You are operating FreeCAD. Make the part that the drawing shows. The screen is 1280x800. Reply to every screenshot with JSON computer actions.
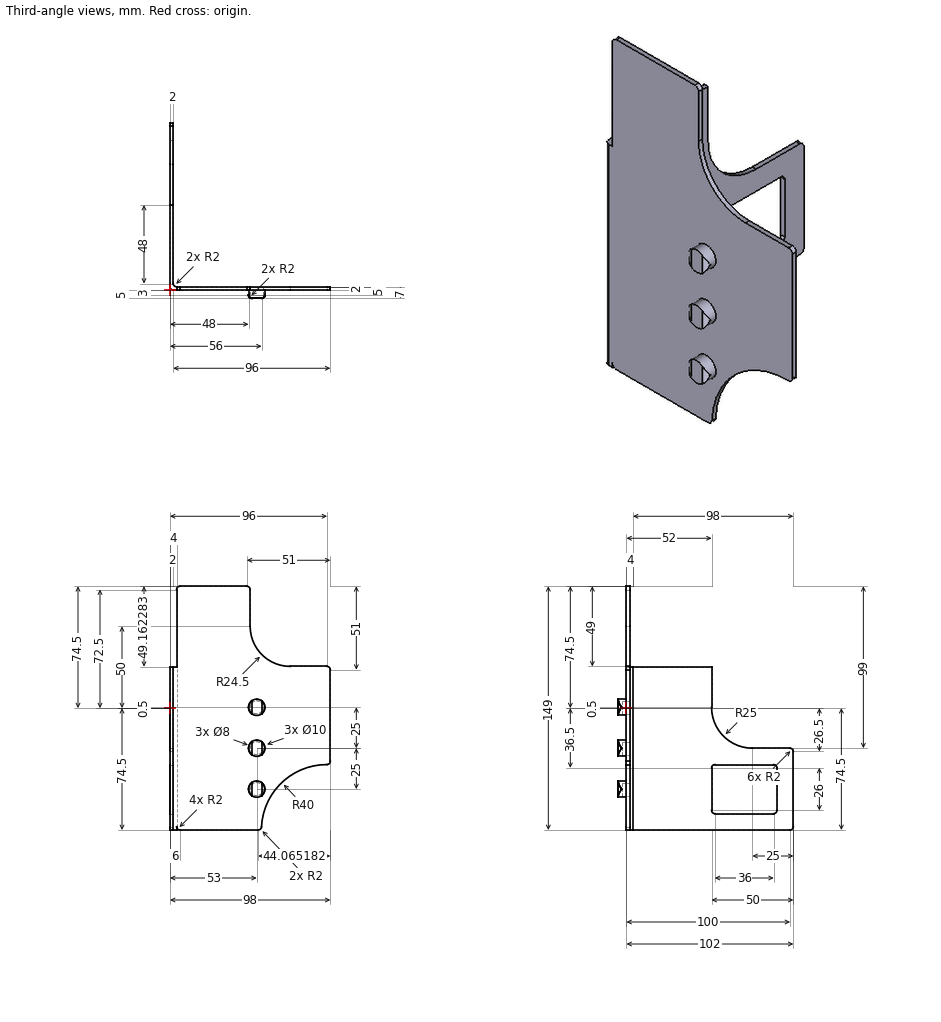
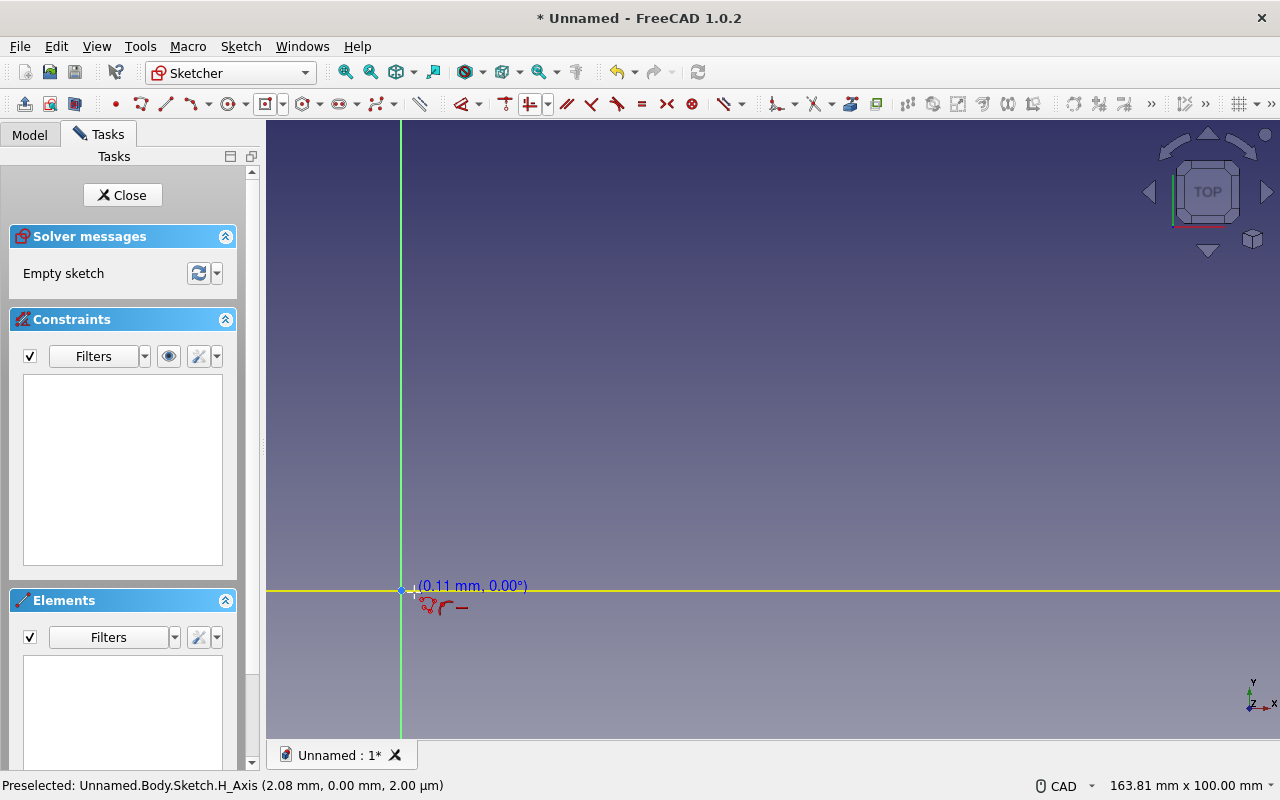
{"action": "left_click", "coordinate": [1008, 582]}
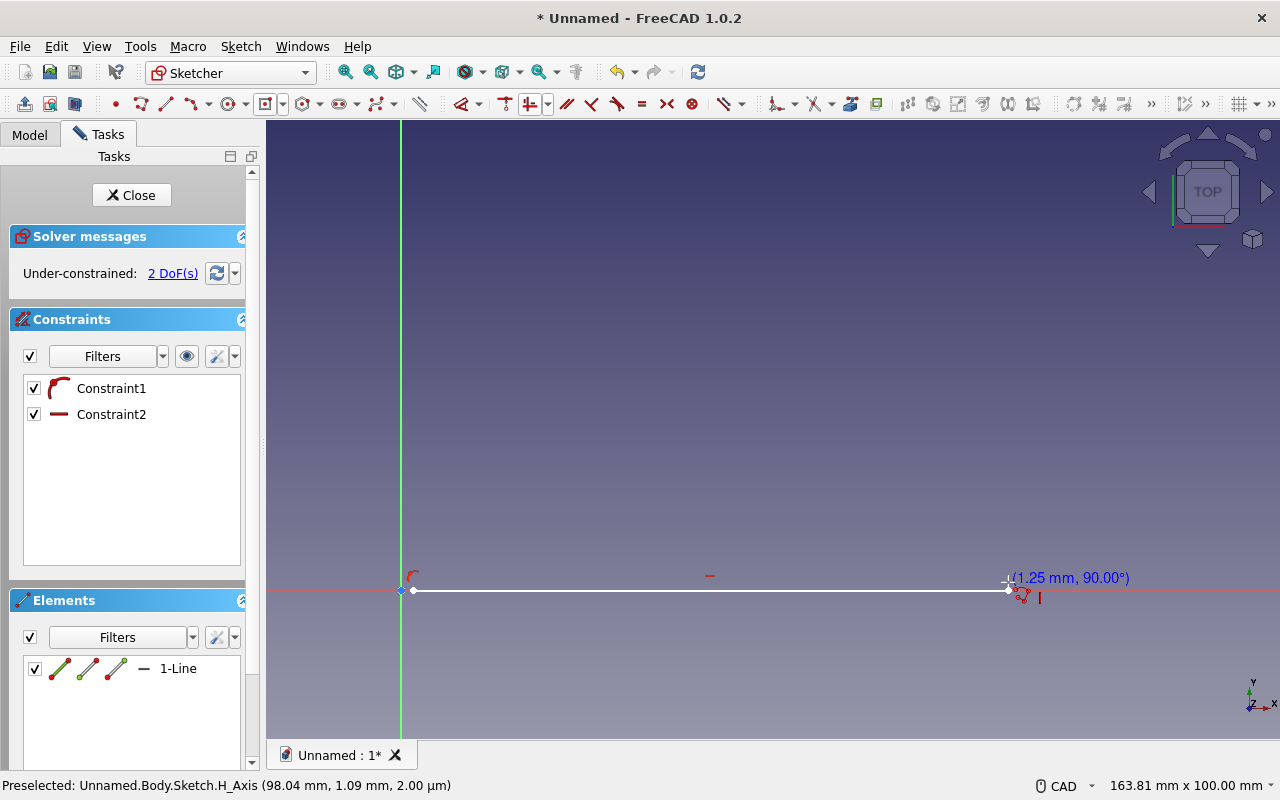
{"action": "scroll", "coordinate": [1008, 578], "scroll_direction": "up", "scroll_amount": 2}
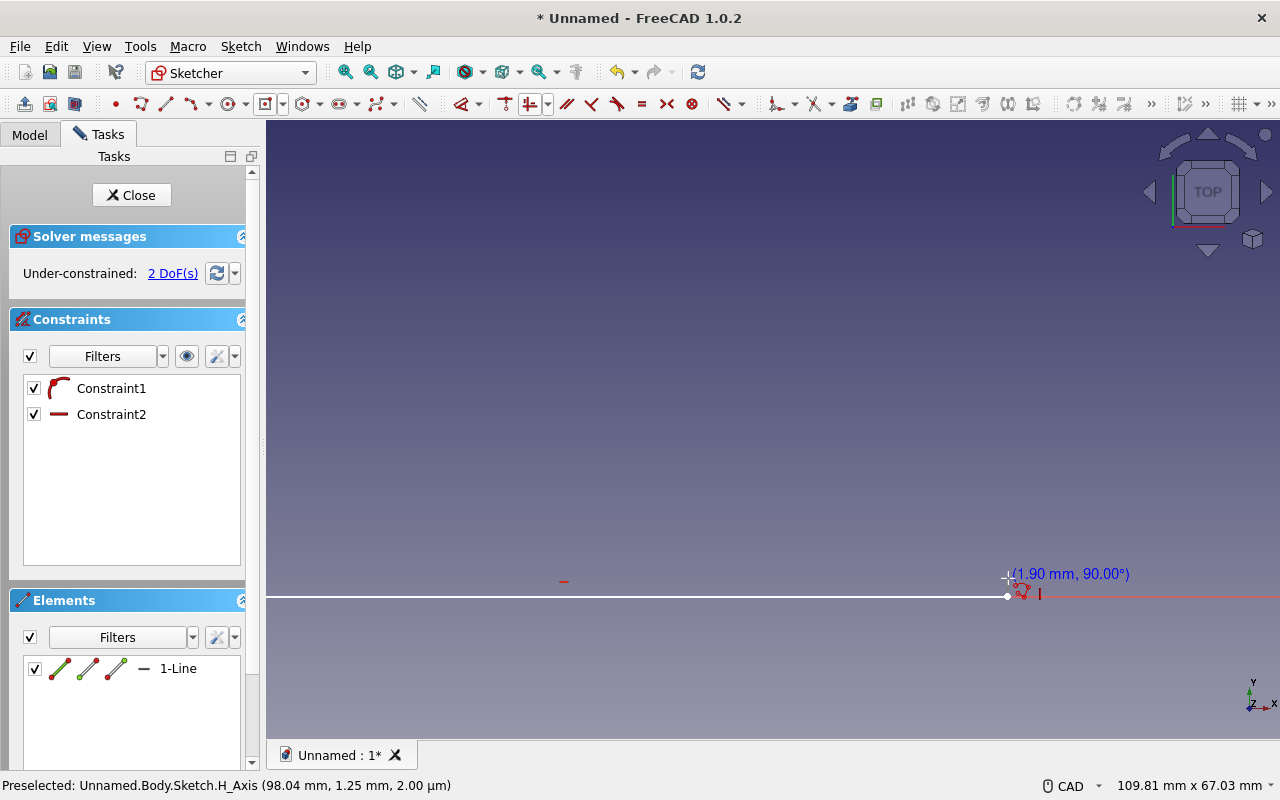
{"action": "left_click", "coordinate": [1008, 578]}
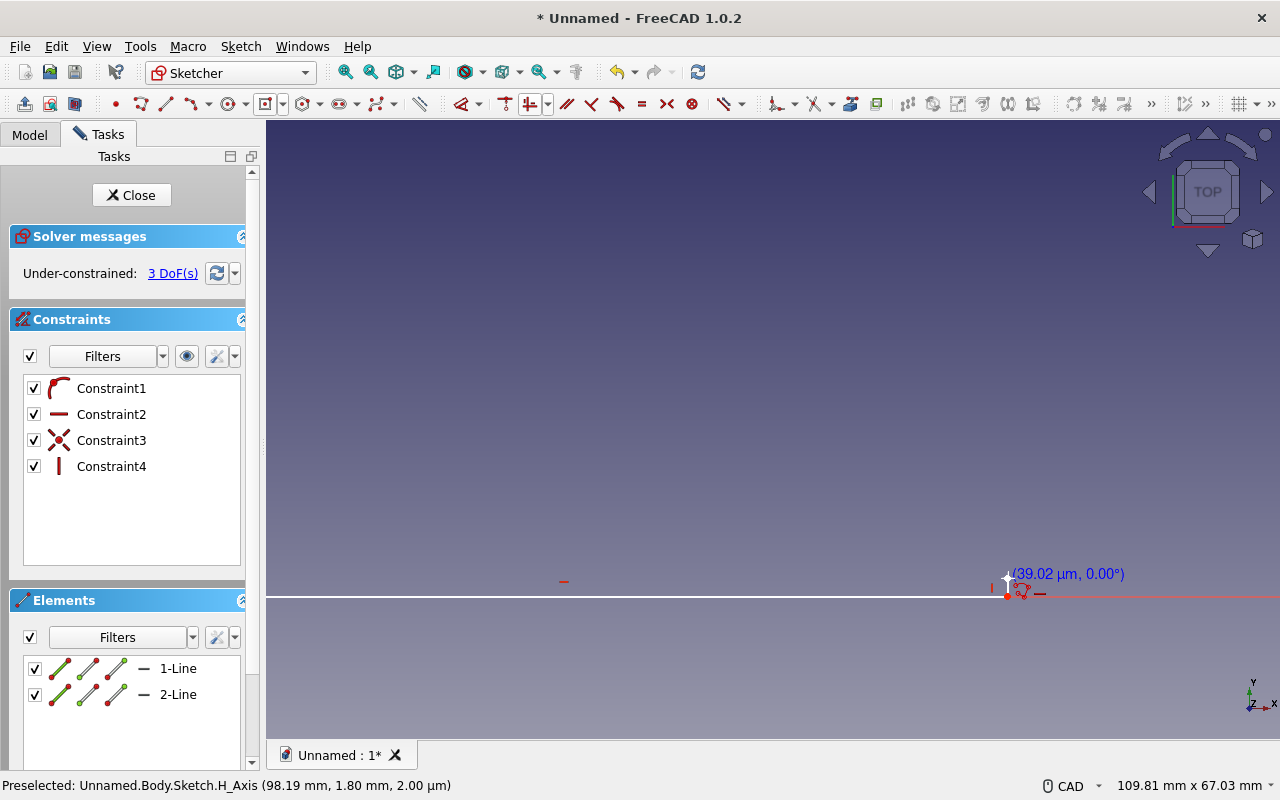
{"action": "scroll", "coordinate": [1009, 578], "scroll_direction": "down", "scroll_amount": 2}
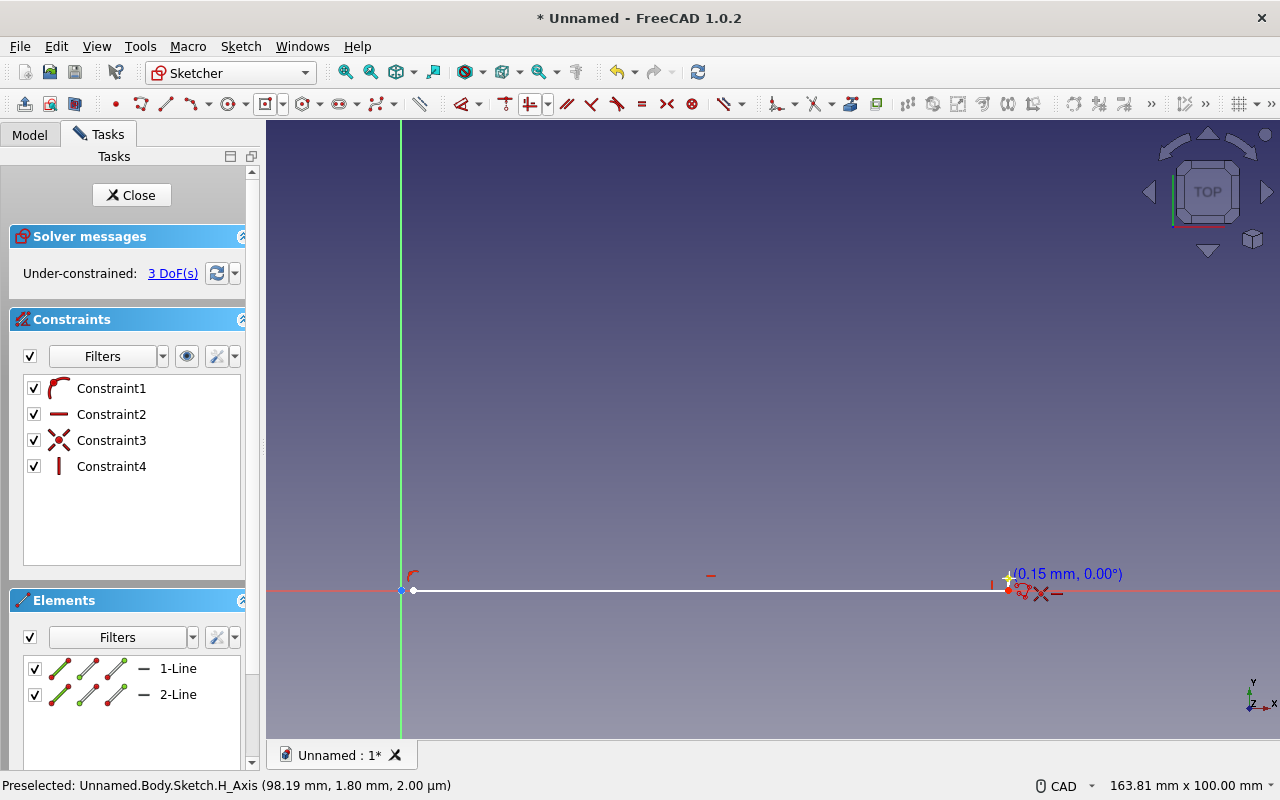
{"action": "scroll", "coordinate": [426, 578], "scroll_direction": "up", "scroll_amount": 2}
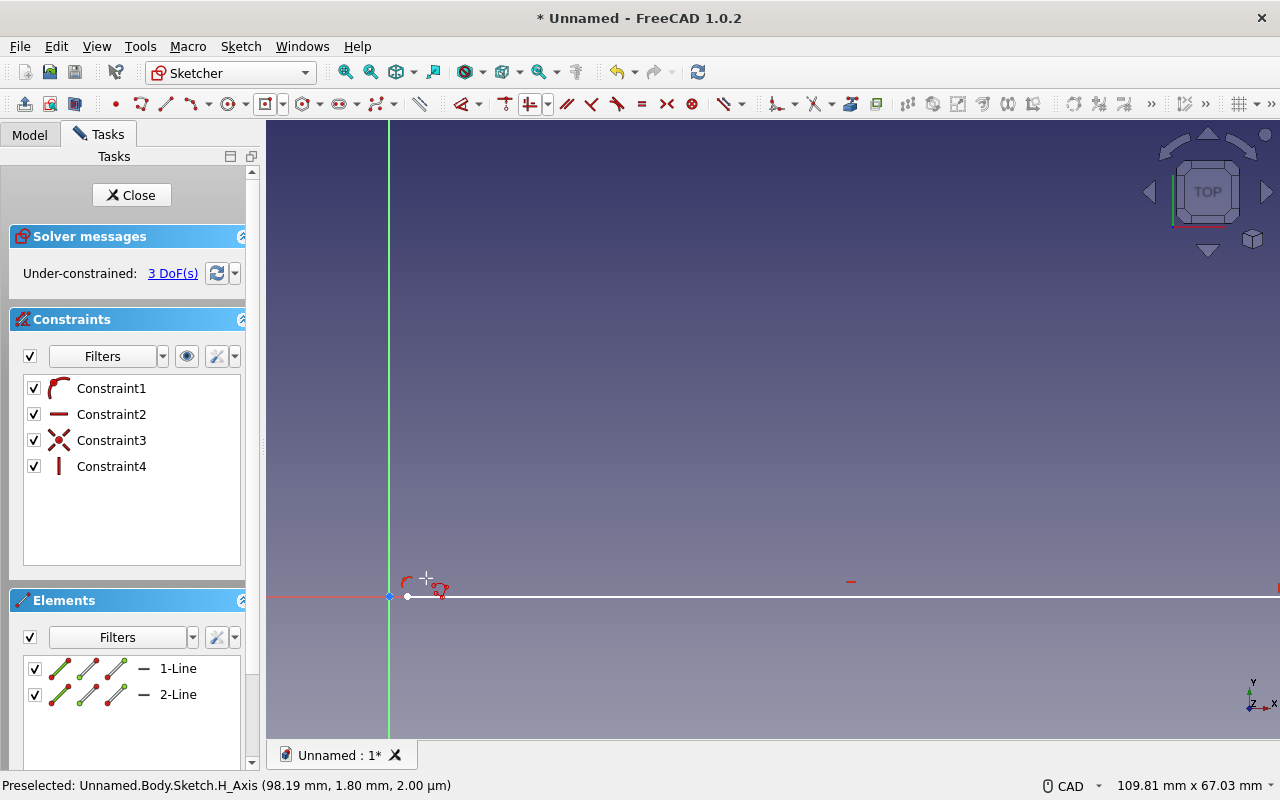
{"action": "left_click", "coordinate": [426, 578]}
{"action": "right_click", "coordinate": [426, 578]}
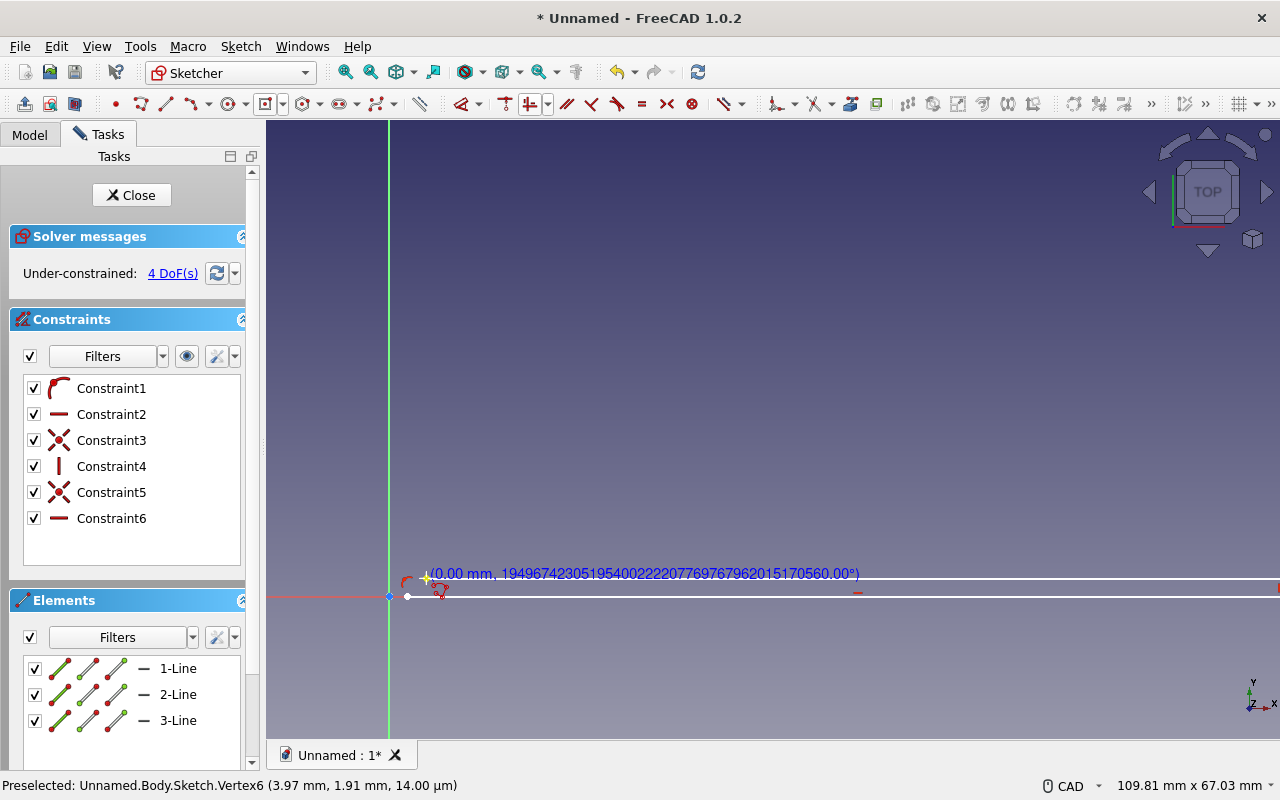
{"action": "left_click", "coordinate": [408, 560]}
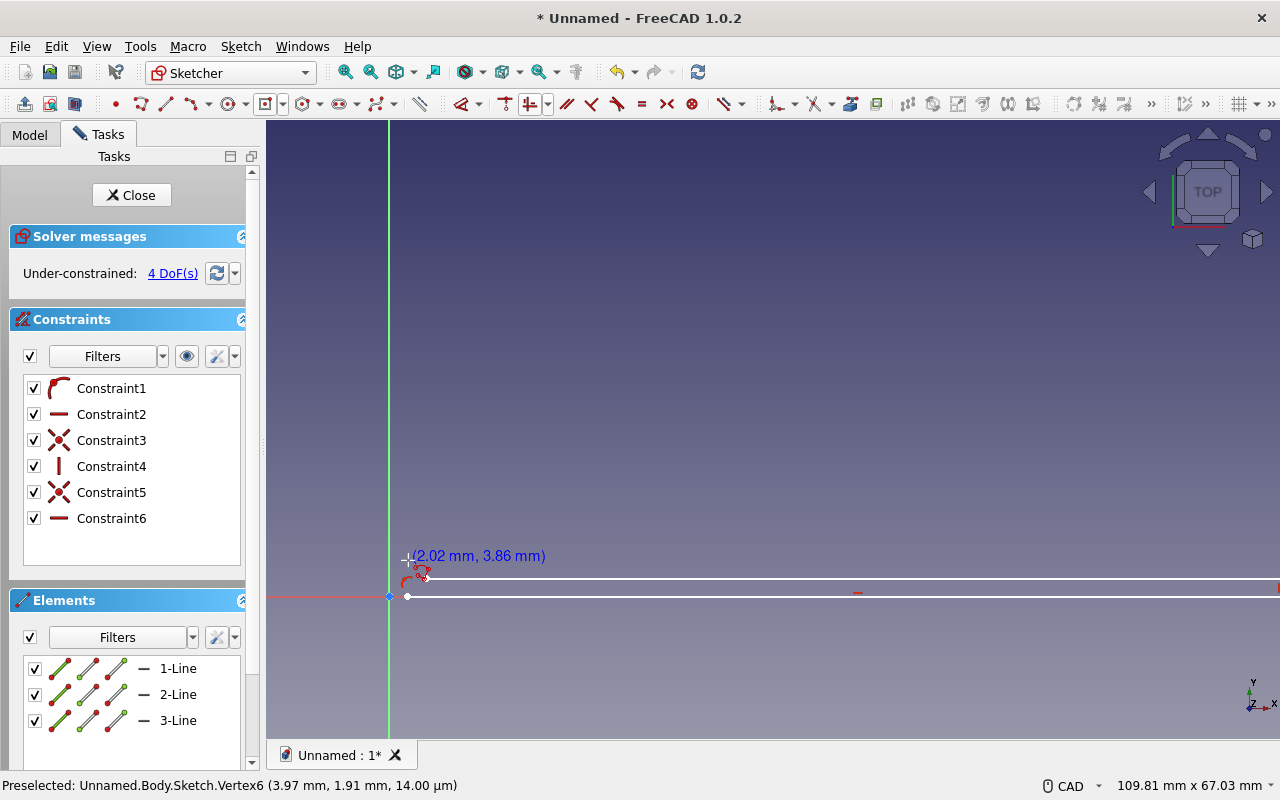
{"action": "scroll", "coordinate": [425, 578], "scroll_direction": "down", "scroll_amount": 2}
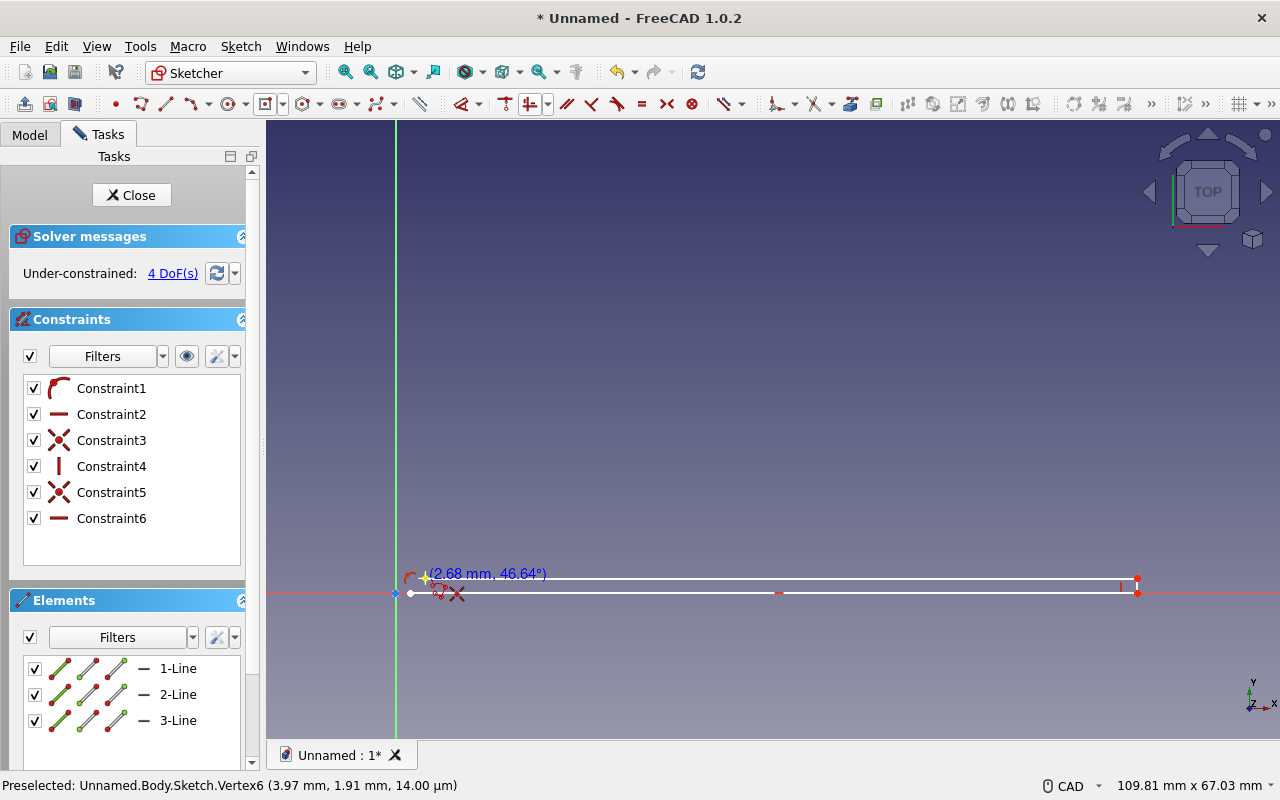
{"action": "scroll", "coordinate": [414, 269], "scroll_direction": "up", "scroll_amount": 2}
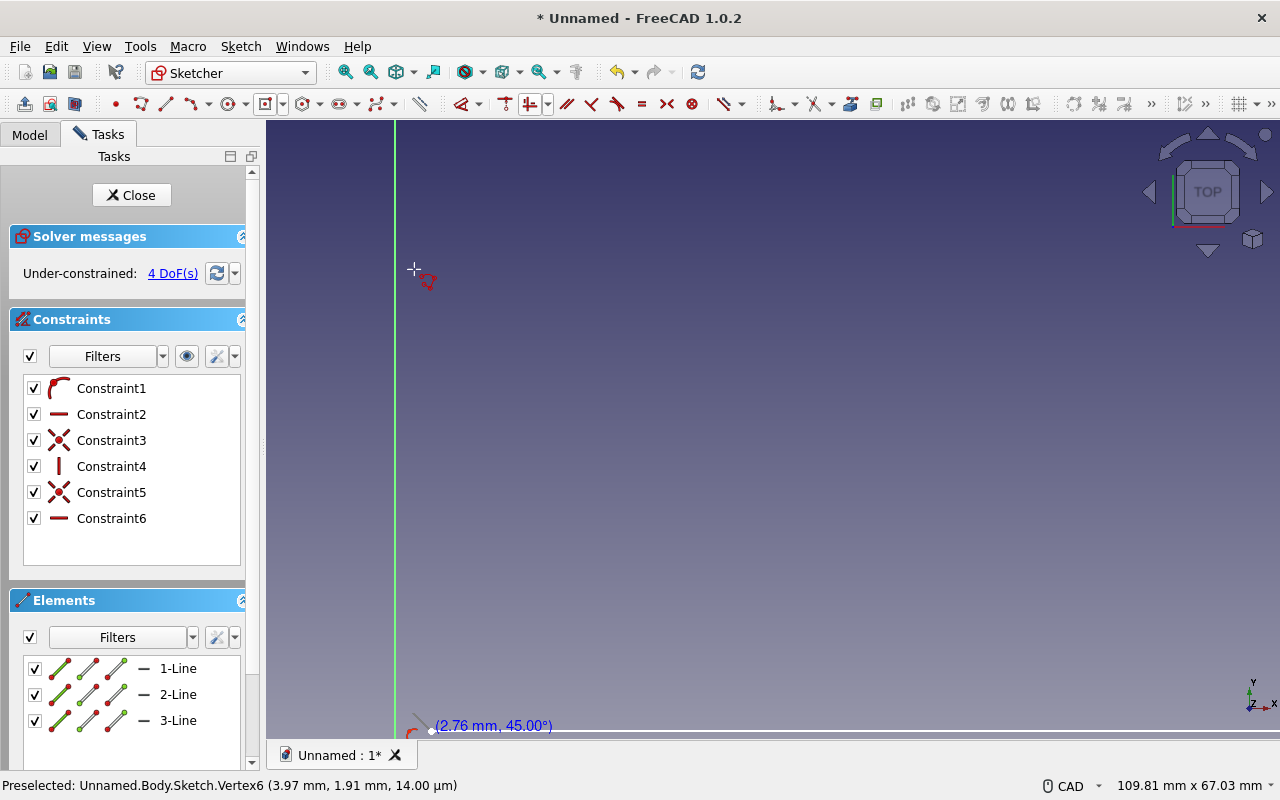
{"action": "left_click", "coordinate": [413, 269]}
{"action": "left_click", "coordinate": [395, 269]}